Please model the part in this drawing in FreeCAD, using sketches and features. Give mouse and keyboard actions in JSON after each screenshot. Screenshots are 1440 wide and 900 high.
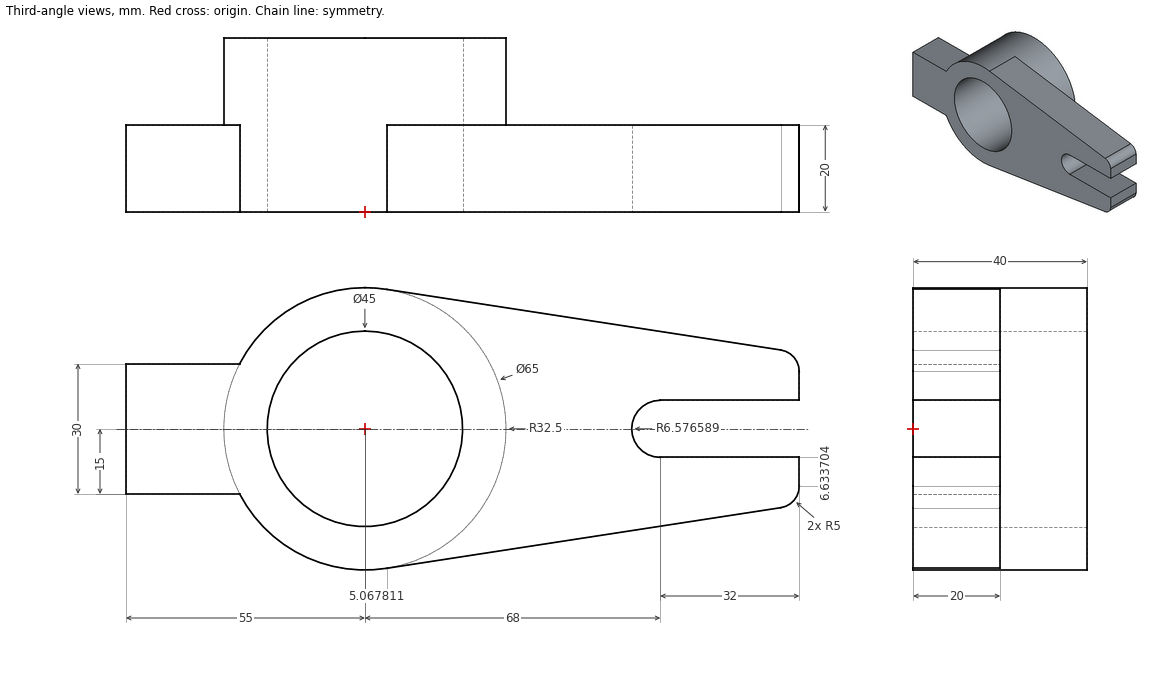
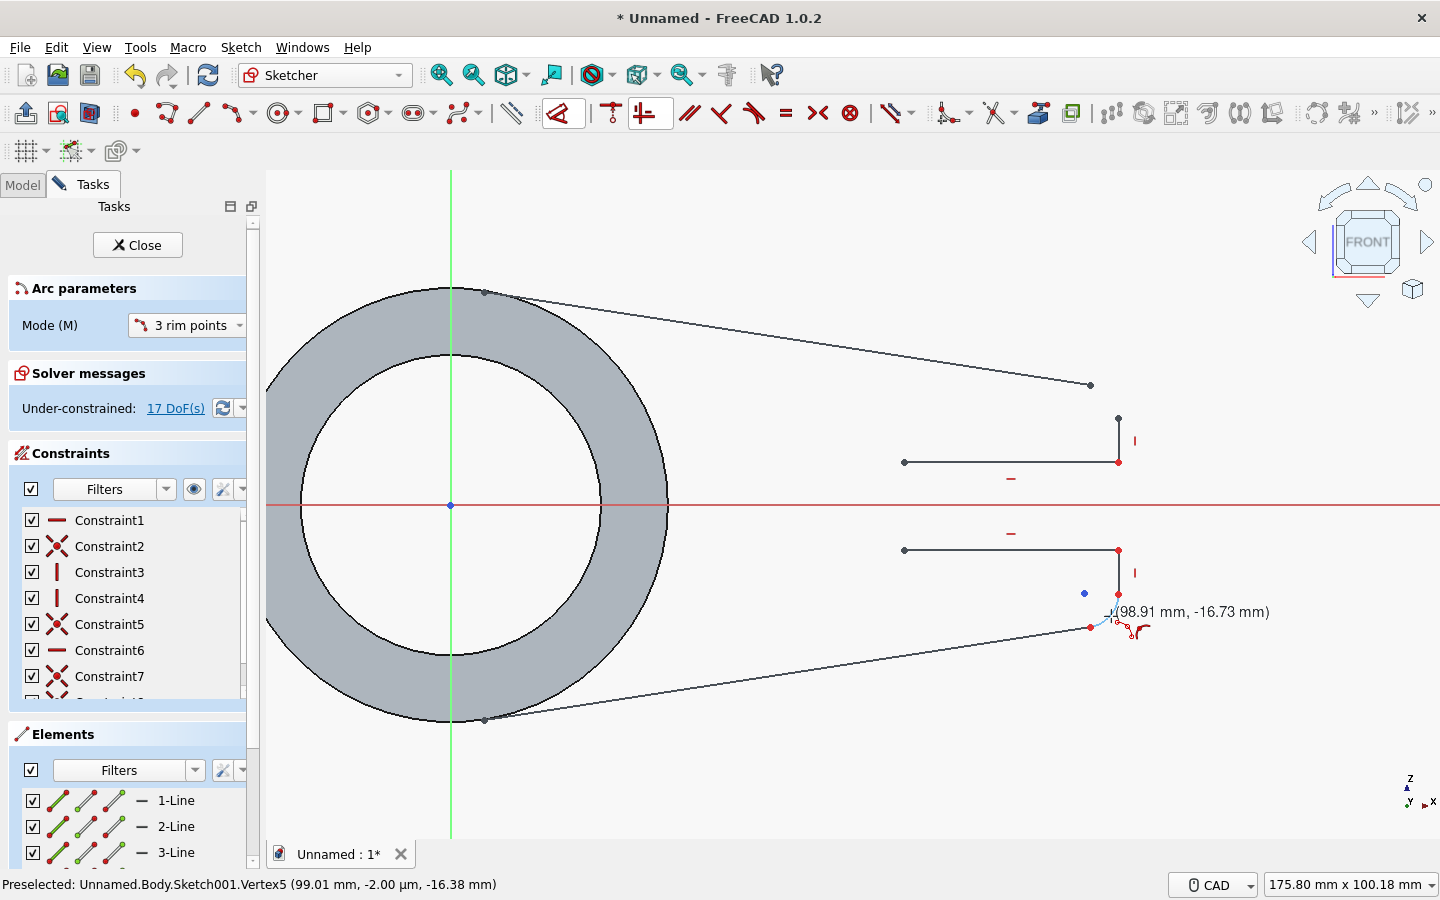
{"action": "left_click", "coordinate": [485, 720]}
{"action": "left_click", "coordinate": [485, 292]}
{"action": "left_click", "coordinate": [659, 566]}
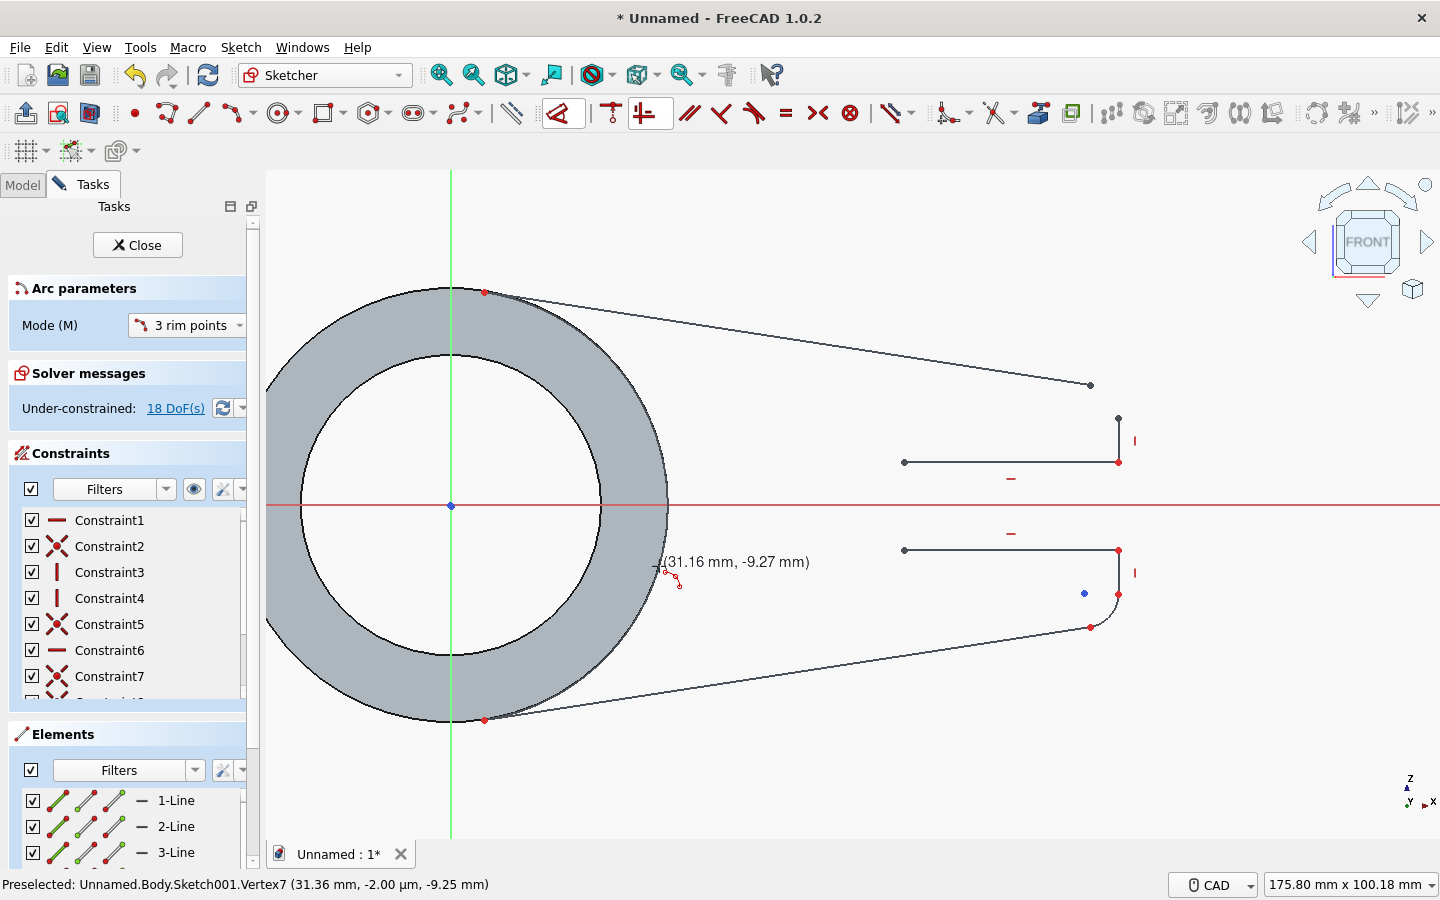
{"action": "left_click", "coordinate": [1091, 385]}
{"action": "left_click", "coordinate": [1119, 418]}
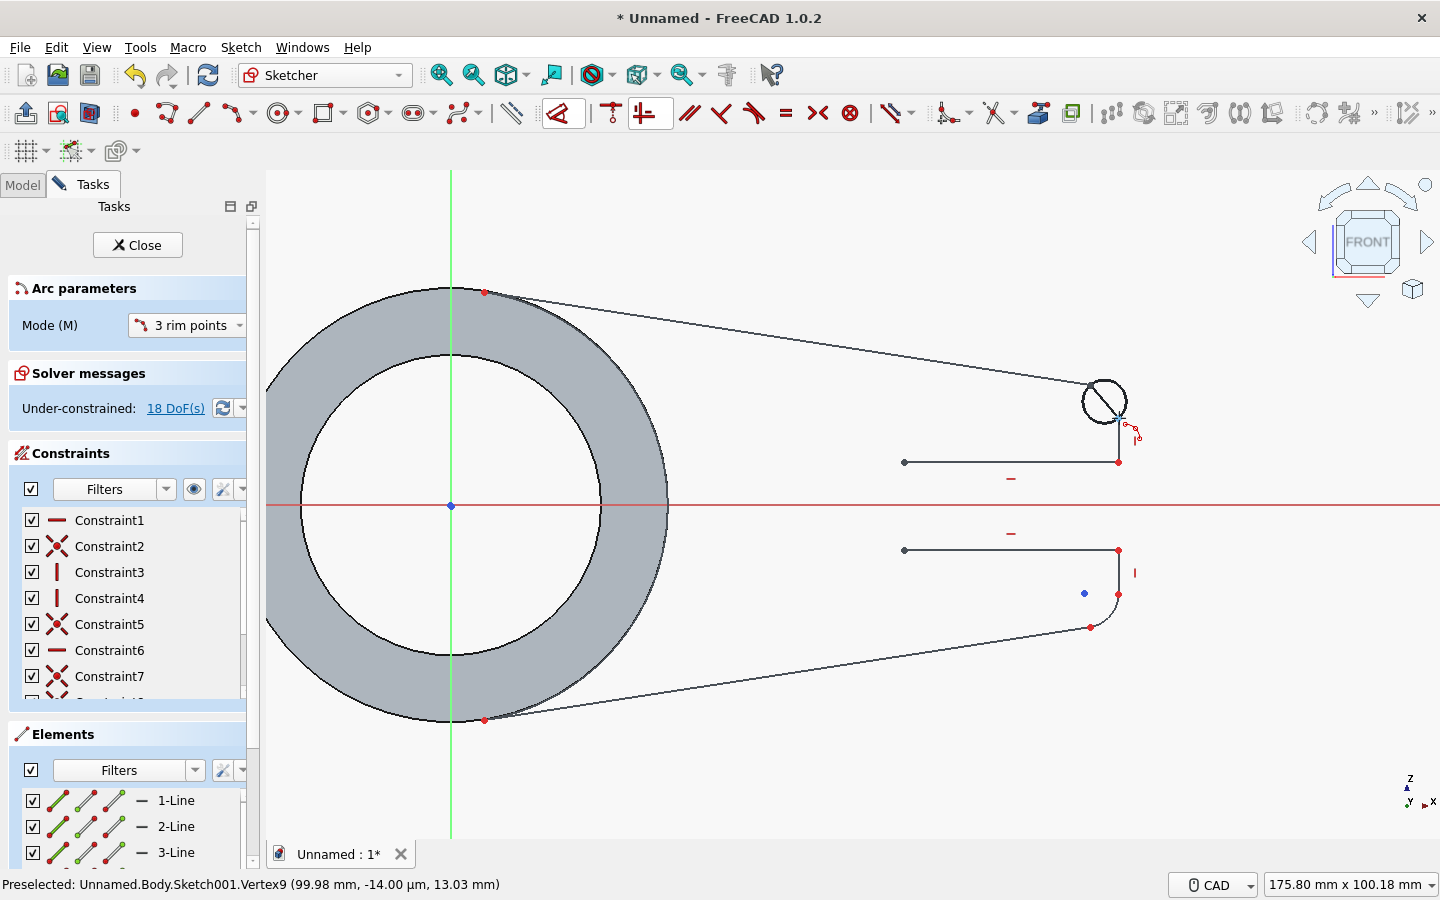
{"action": "scroll", "coordinate": [1111, 395], "scroll_direction": "up", "scroll_amount": 4}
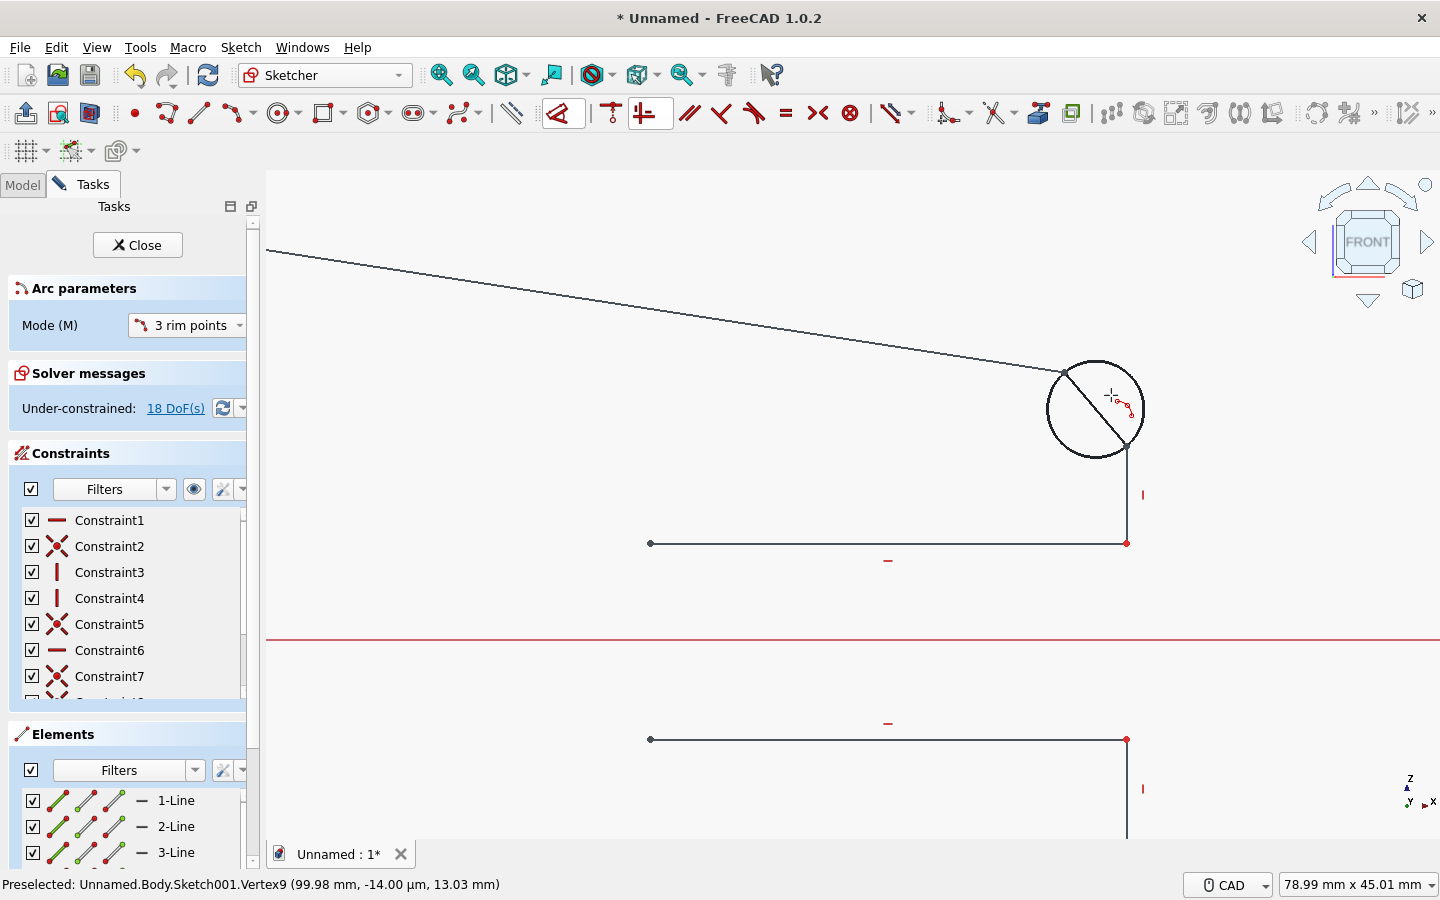
{"action": "left_click", "coordinate": [1109, 395]}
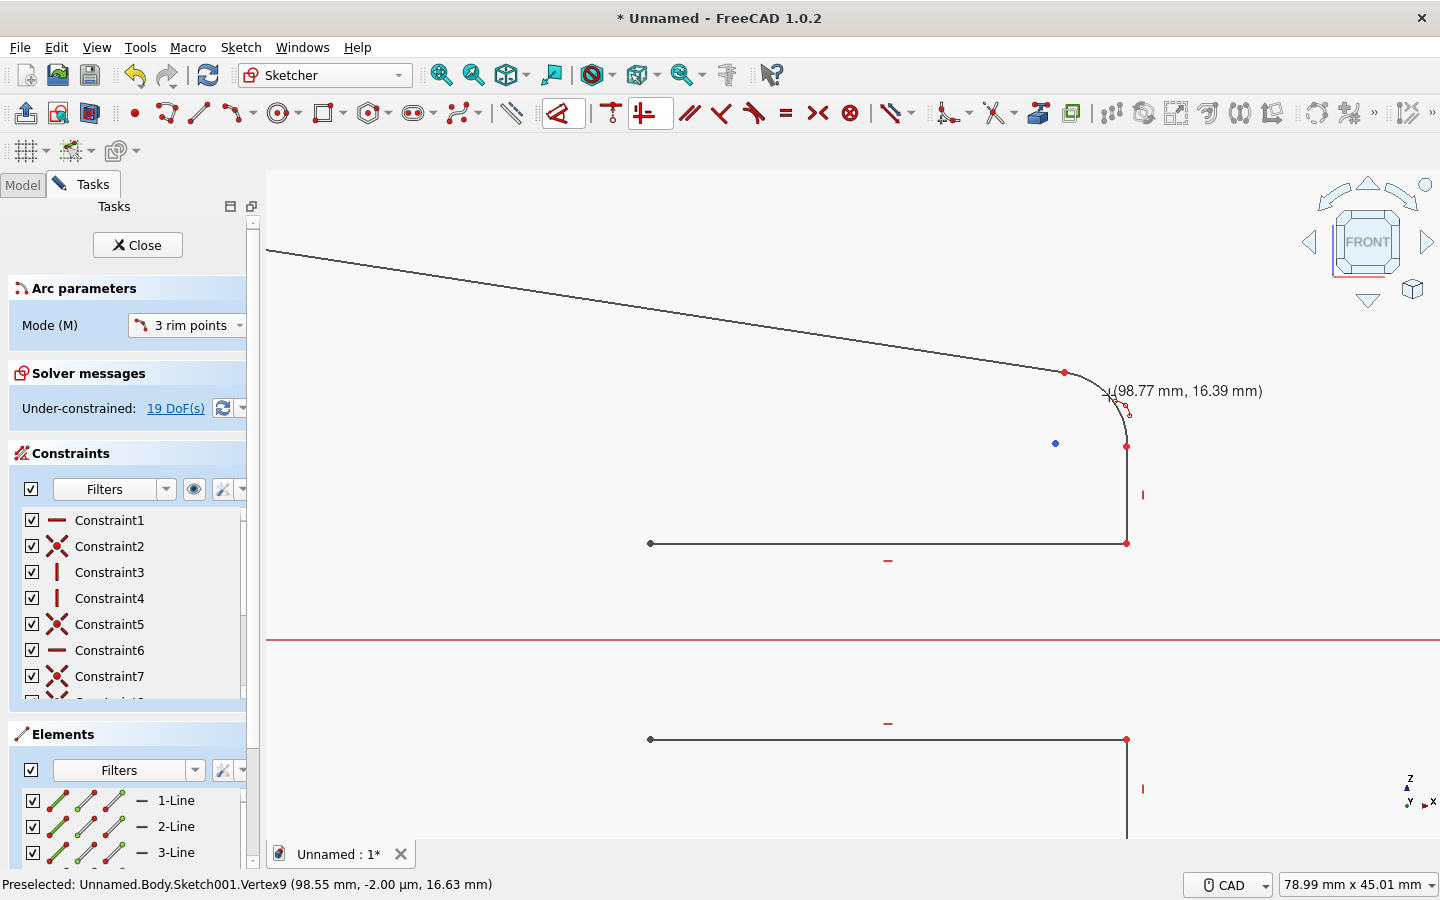
{"action": "left_click", "coordinate": [651, 544]}
{"action": "left_click", "coordinate": [651, 740]}
{"action": "left_click", "coordinate": [573, 582]}
{"action": "key", "text": "Escape"}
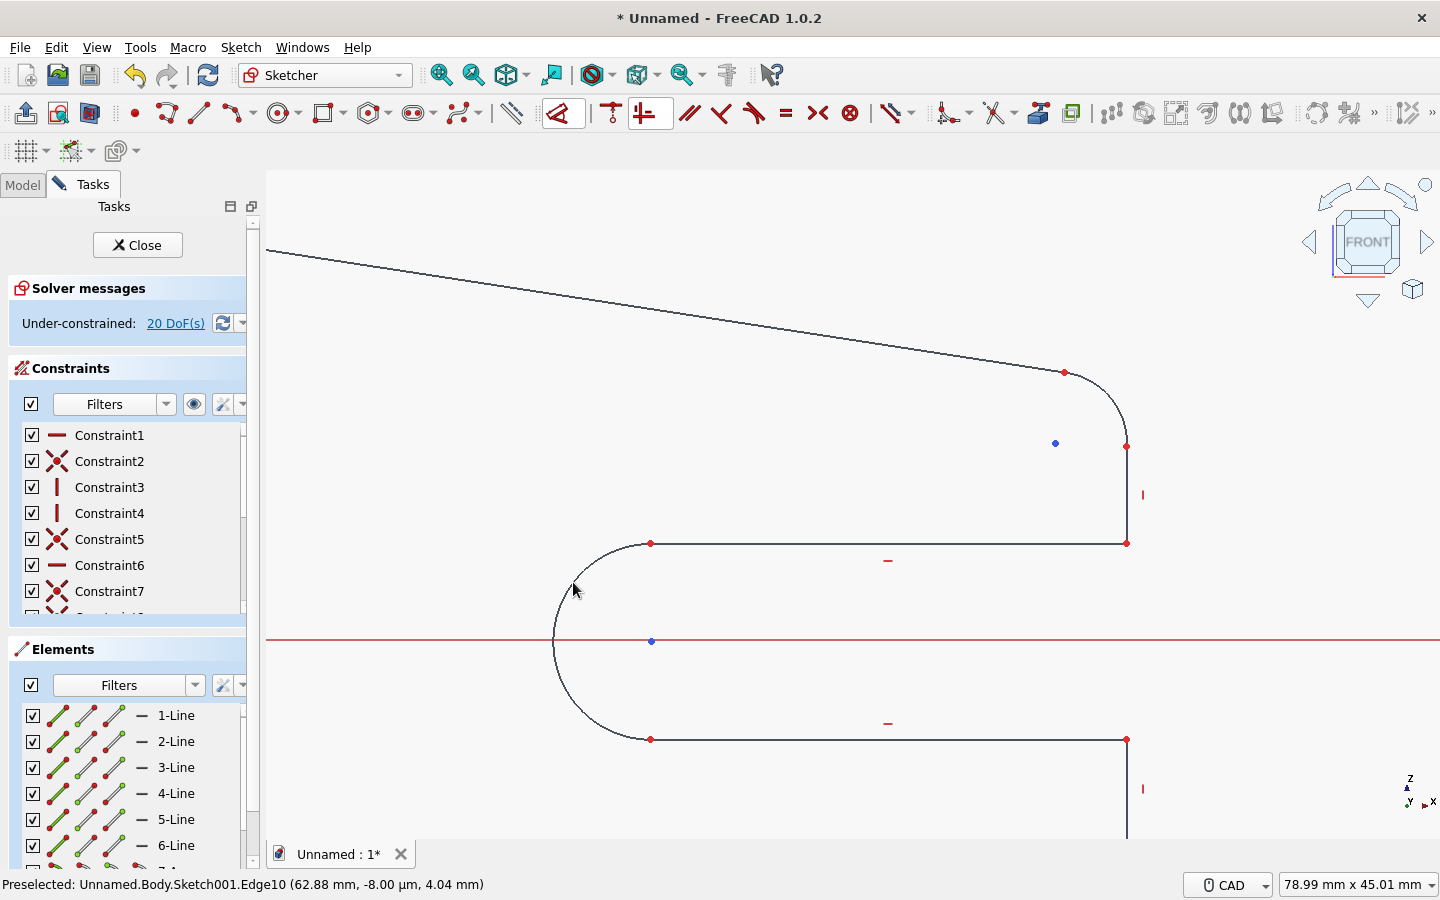
{"action": "left_click", "coordinate": [794, 740]}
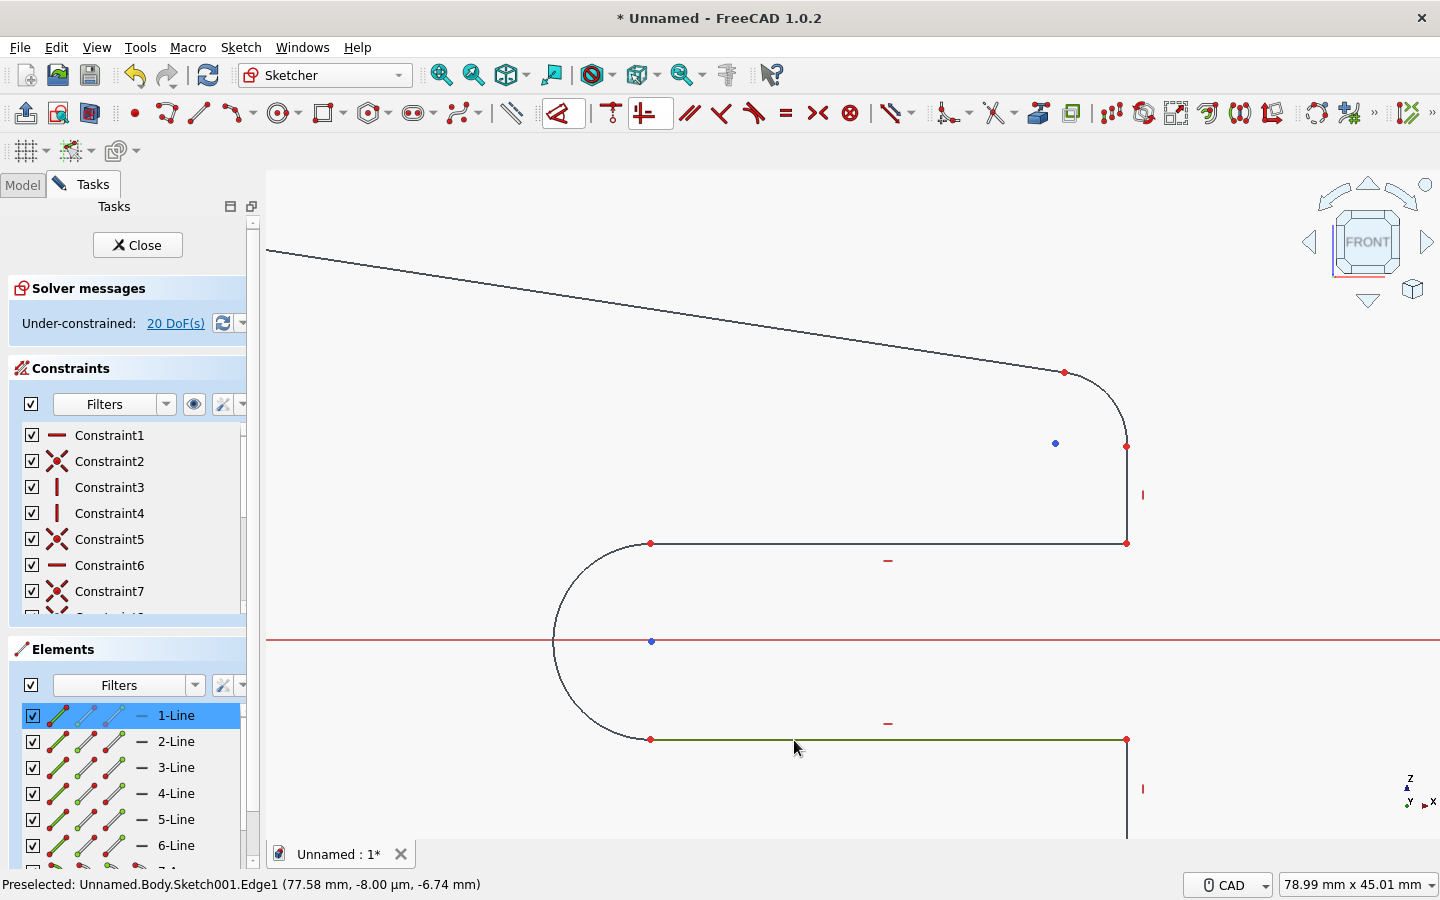
{"action": "left_click", "coordinate": [572, 584]}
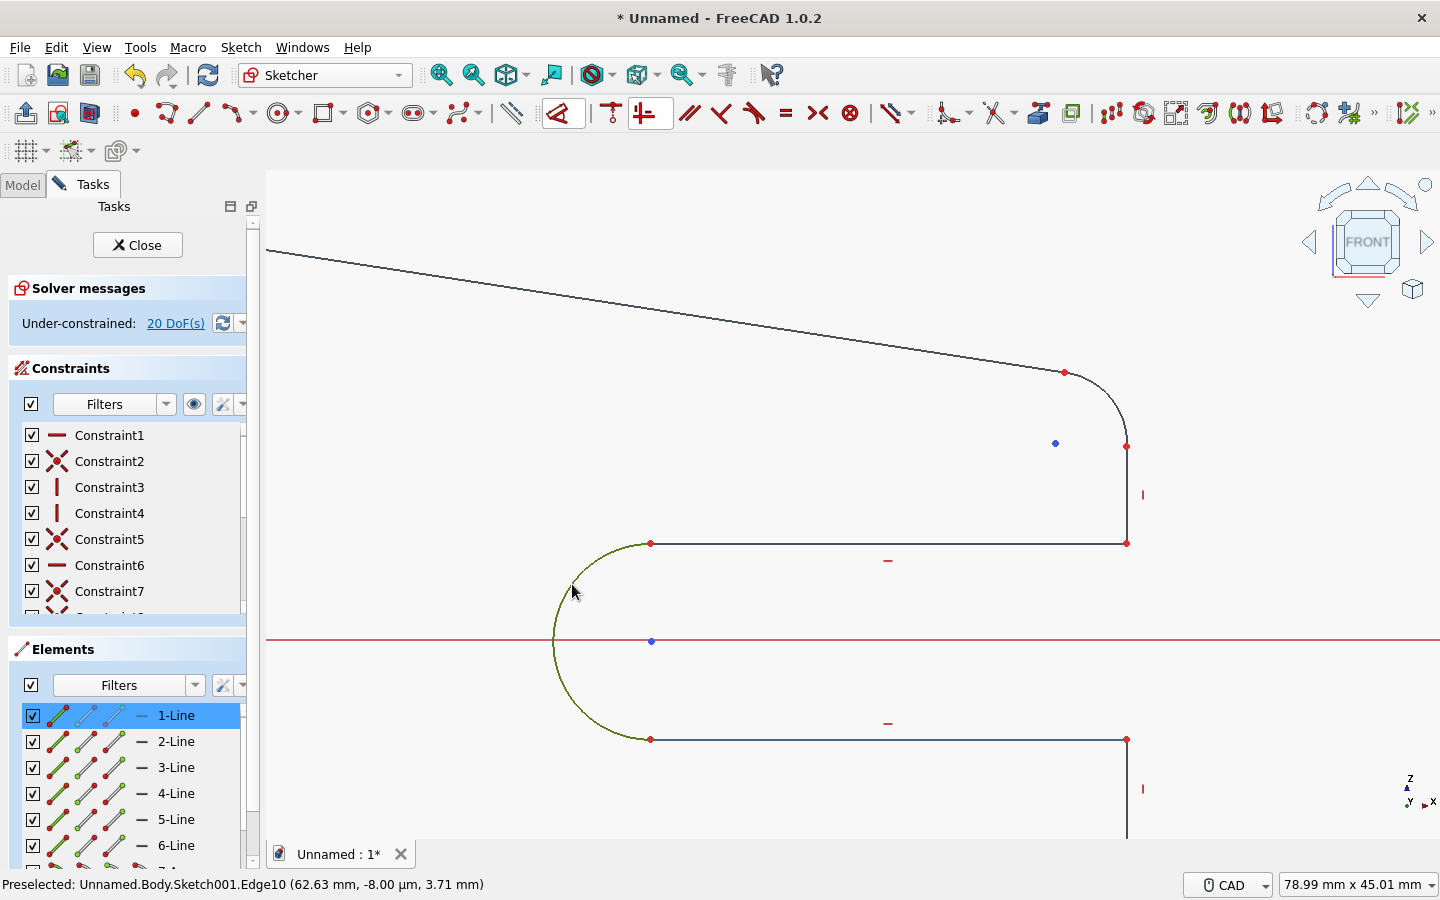
{"action": "left_click", "coordinate": [754, 114]}